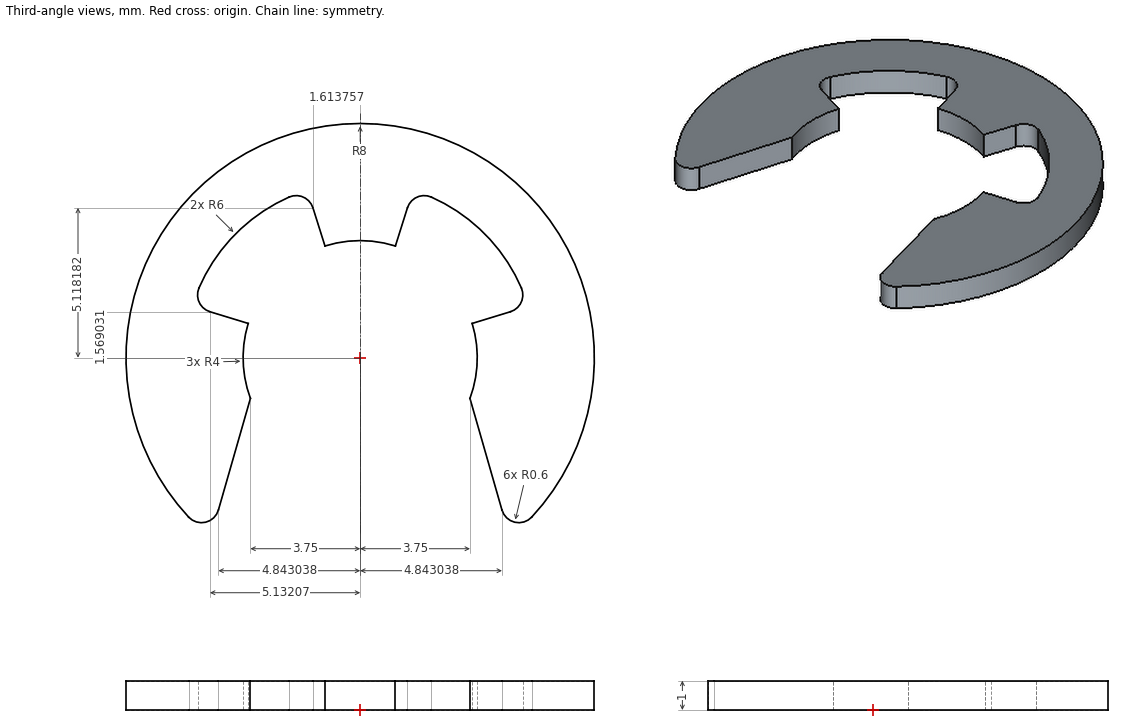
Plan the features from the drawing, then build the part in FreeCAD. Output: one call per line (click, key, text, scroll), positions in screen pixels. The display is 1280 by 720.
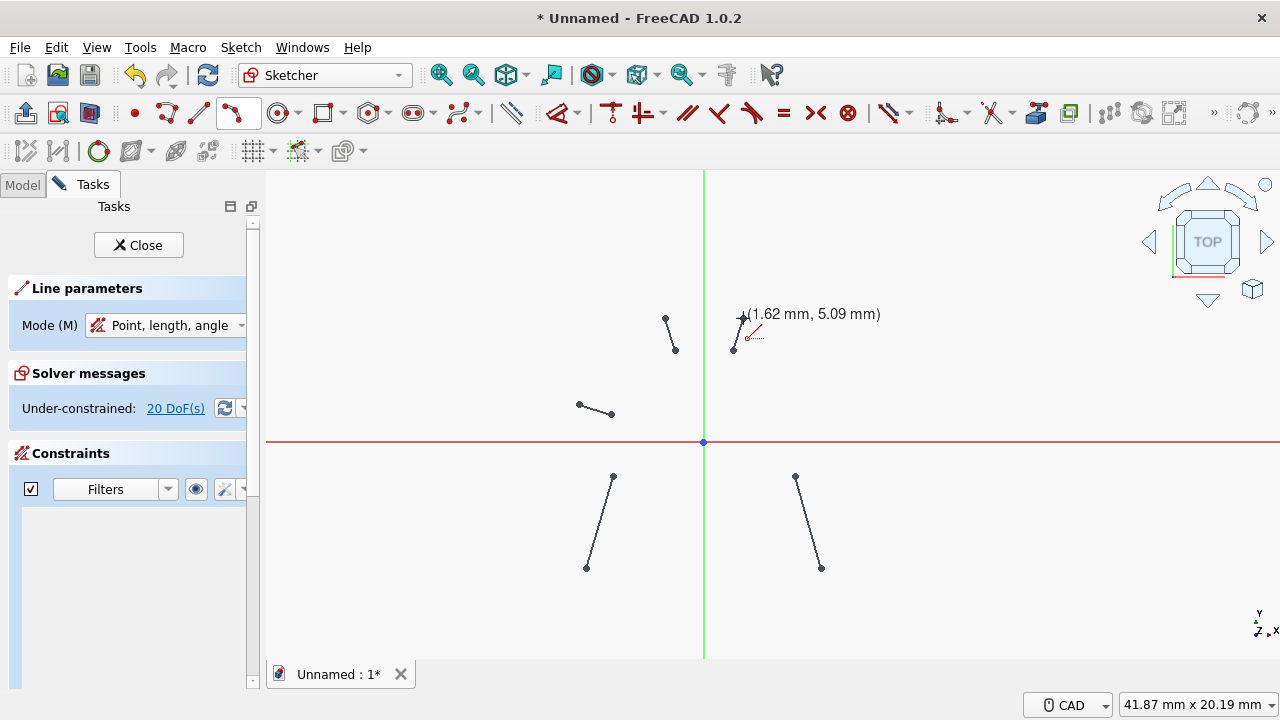
click(828, 404)
click(796, 414)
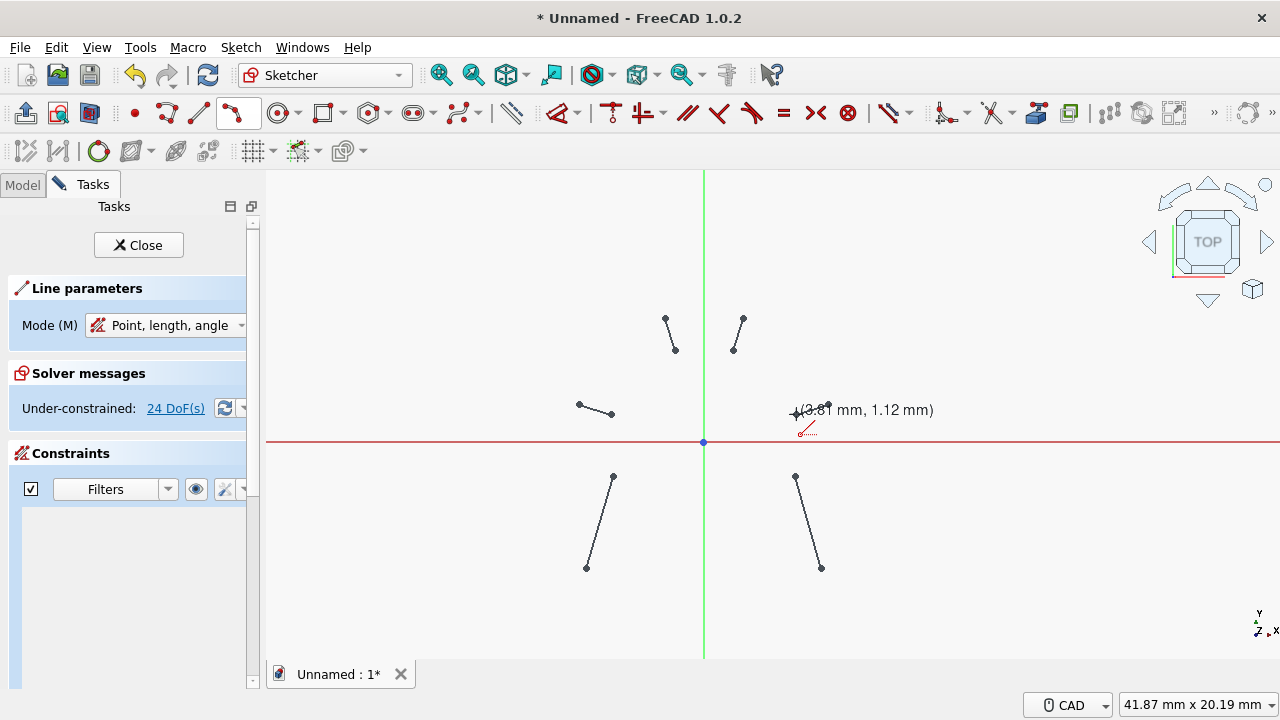
click(232, 114)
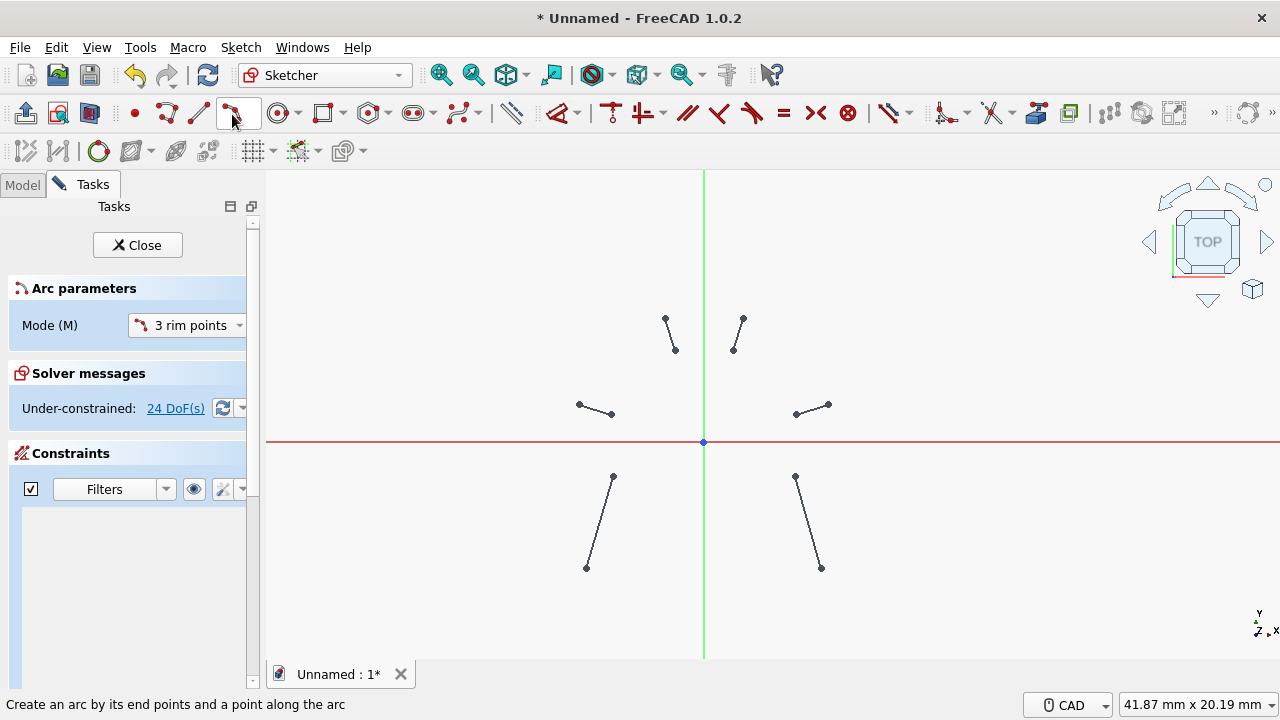
click(821, 569)
click(846, 574)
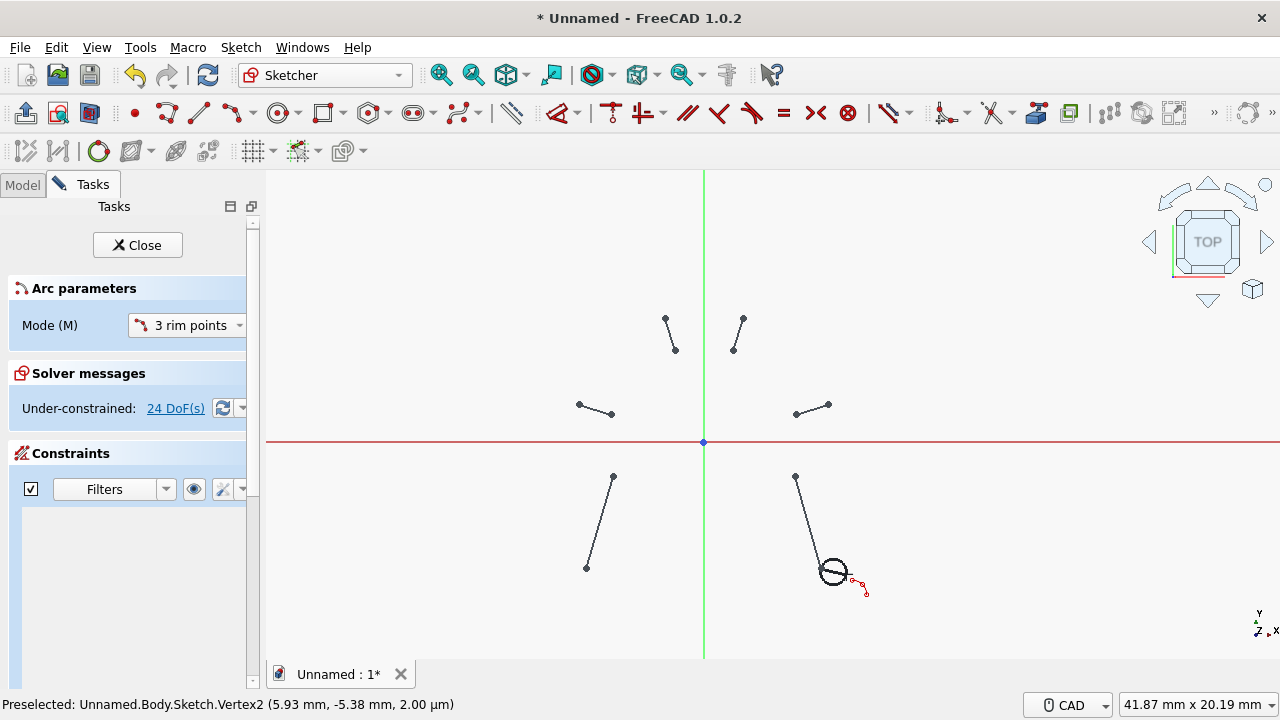
scroll(832, 578, up, 4)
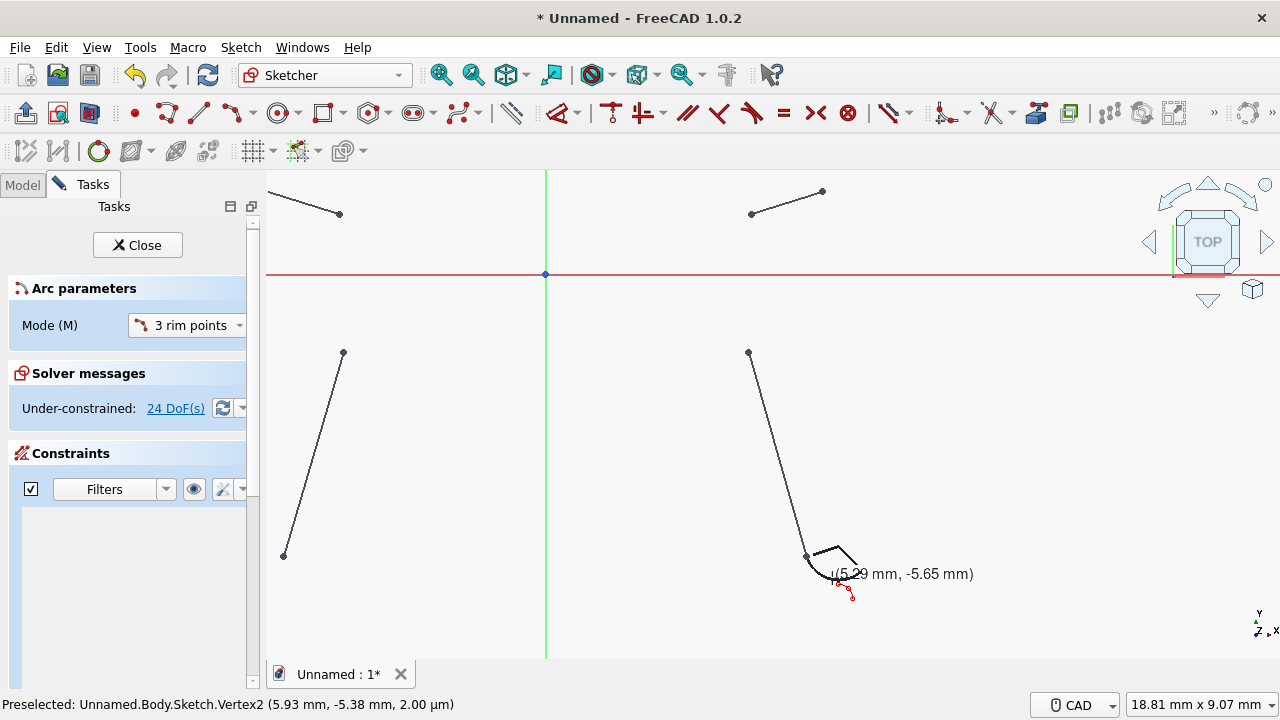
click(831, 578)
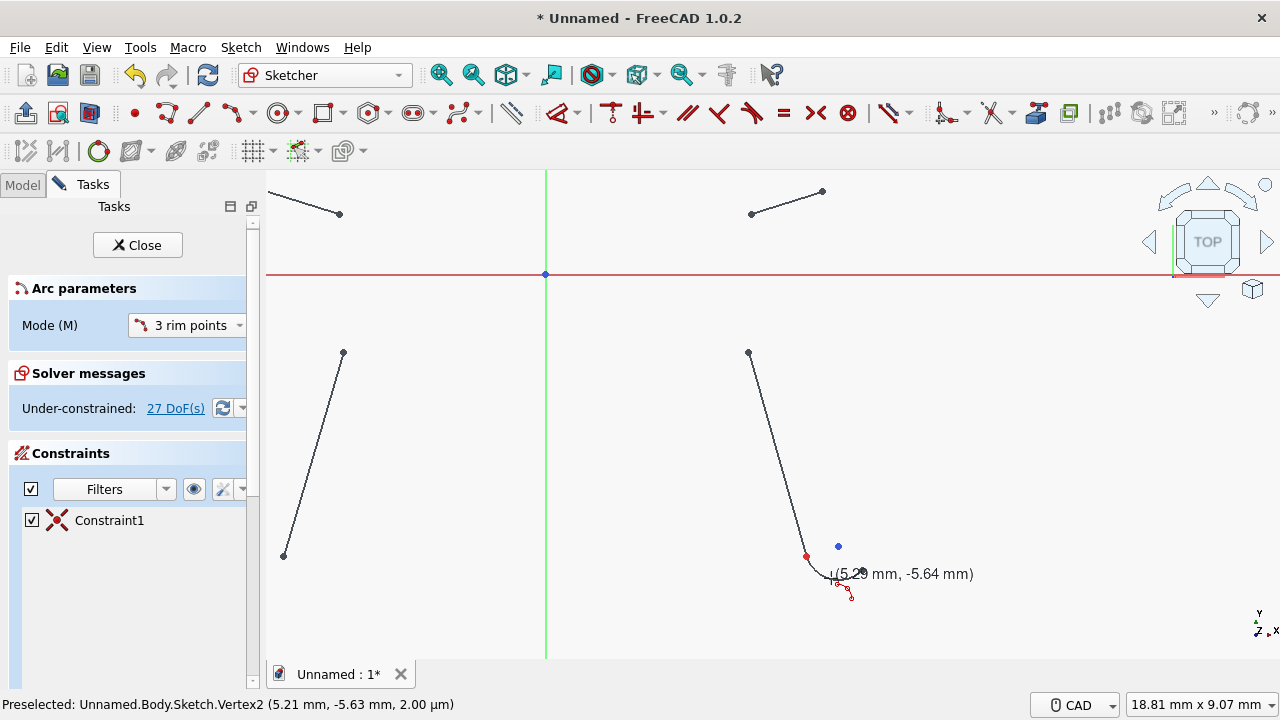
click(862, 570)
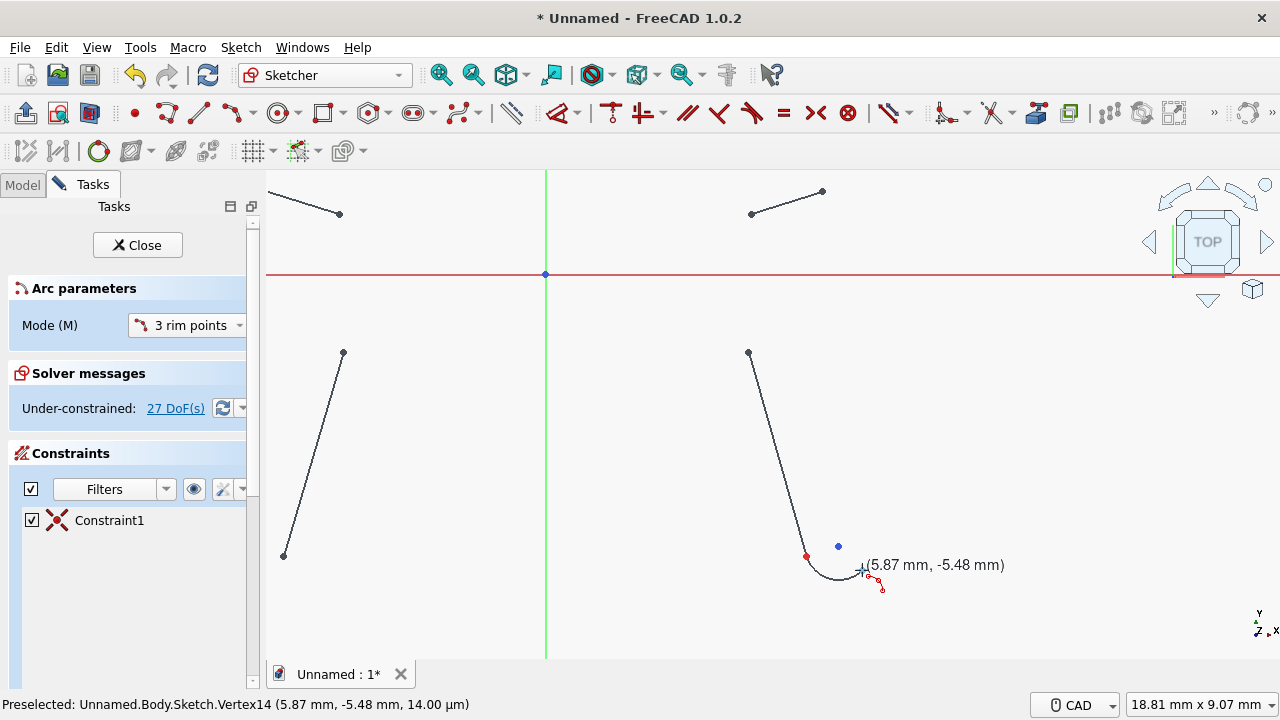
scroll(834, 581, down, 4)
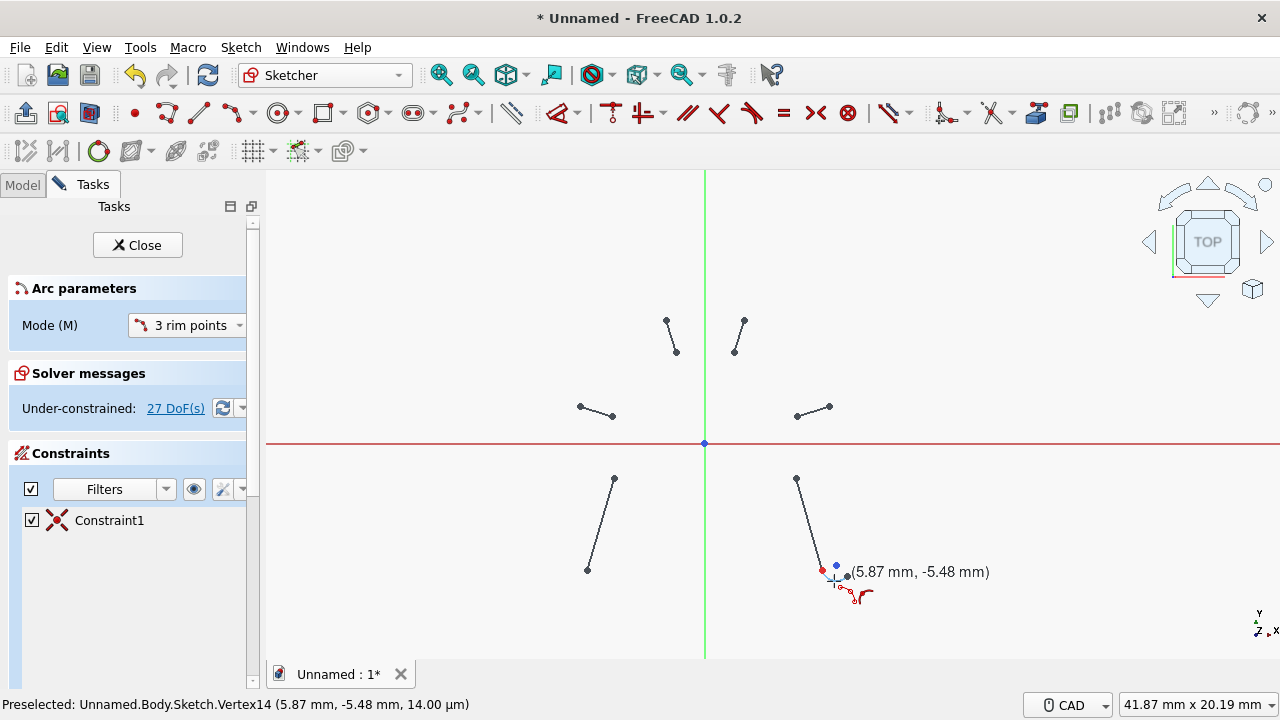
click(563, 576)
click(792, 271)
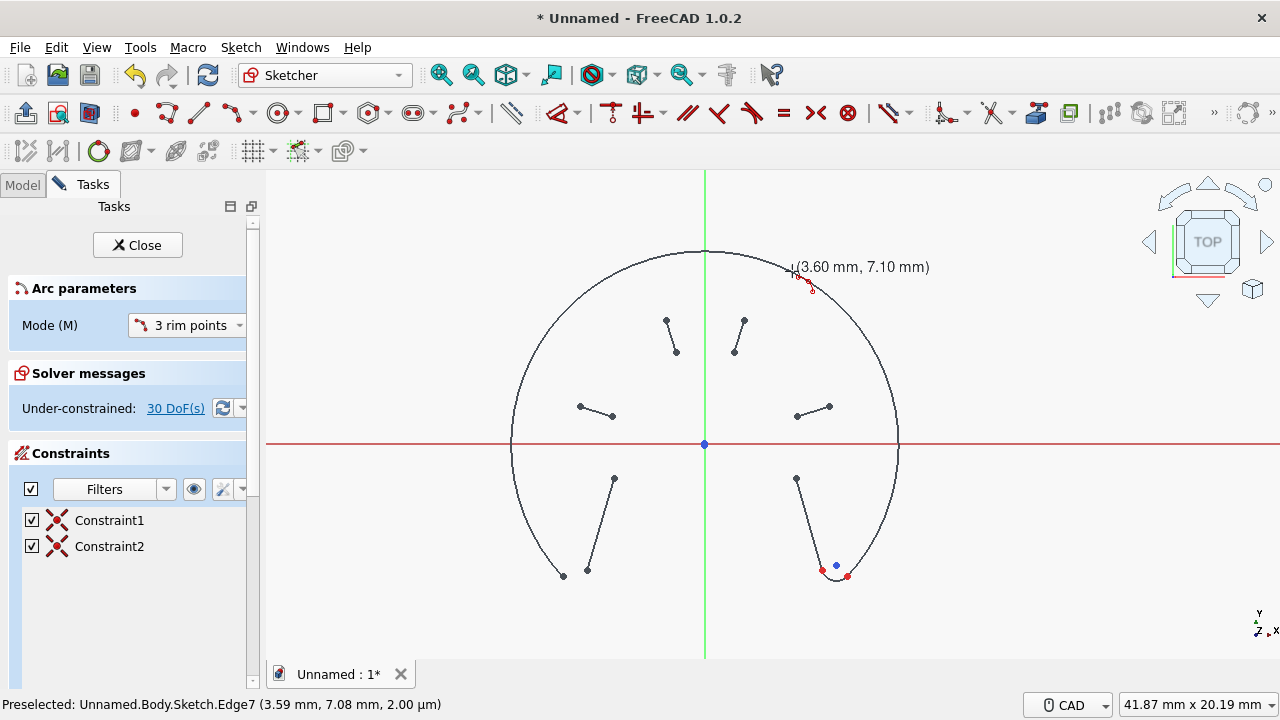
click(563, 577)
click(587, 571)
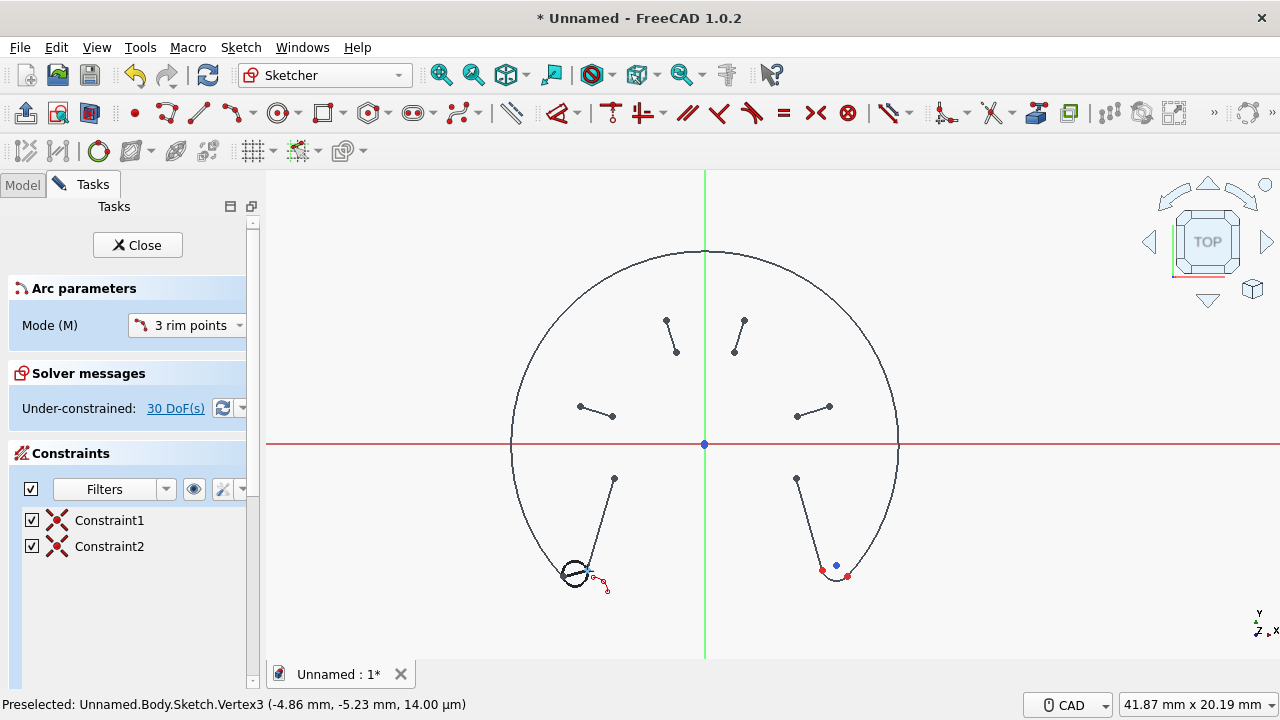
scroll(577, 580, up, 4)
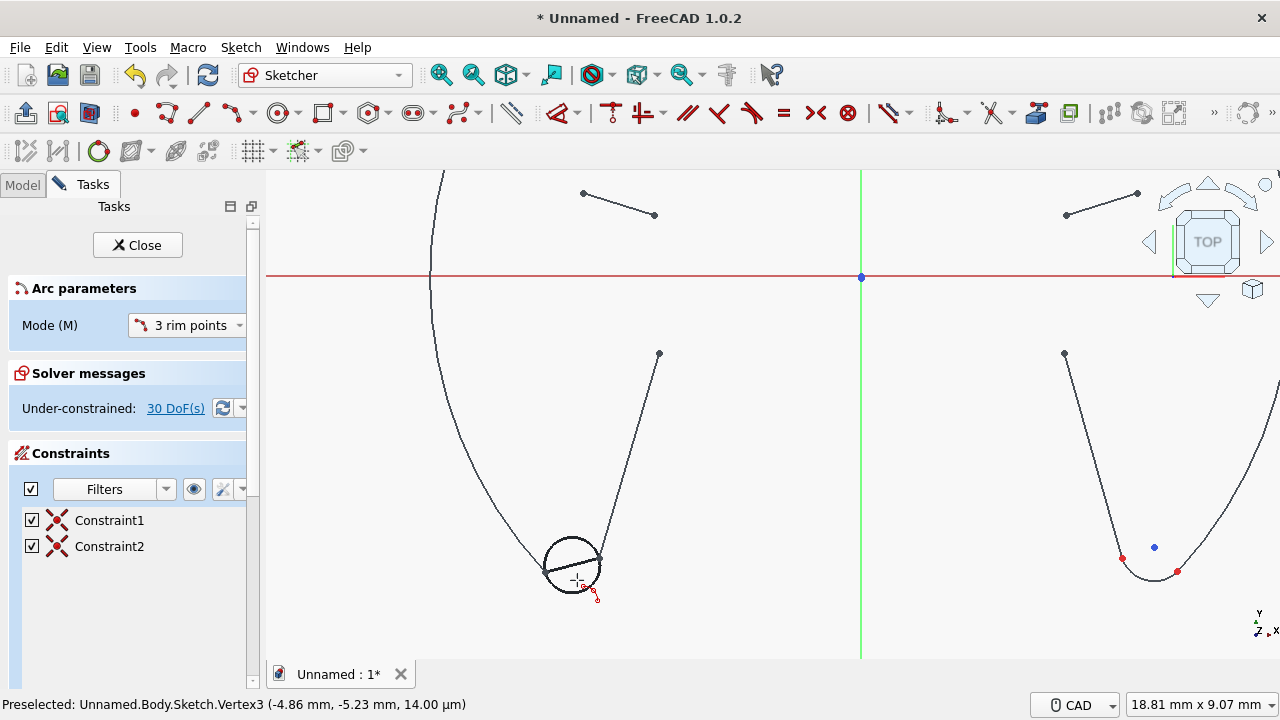
click(577, 579)